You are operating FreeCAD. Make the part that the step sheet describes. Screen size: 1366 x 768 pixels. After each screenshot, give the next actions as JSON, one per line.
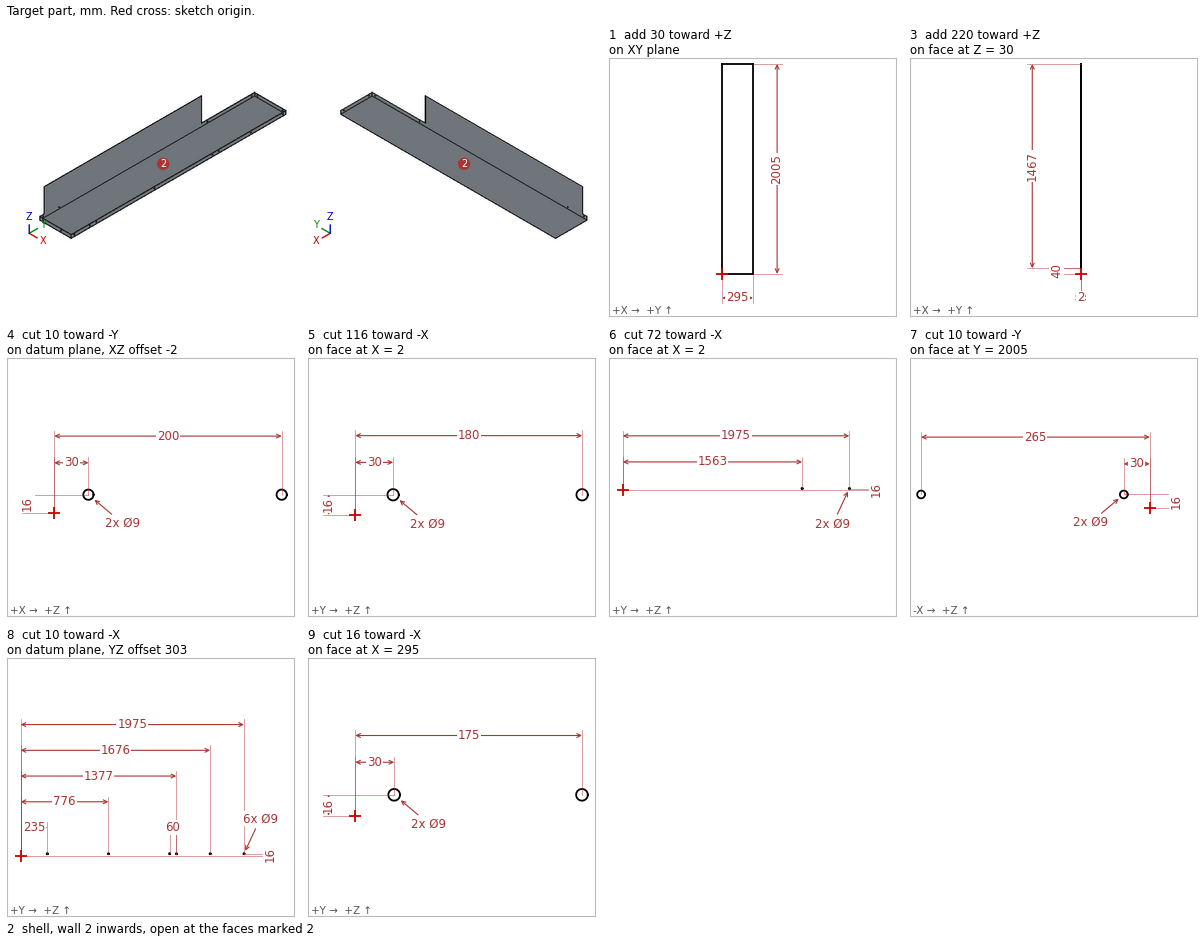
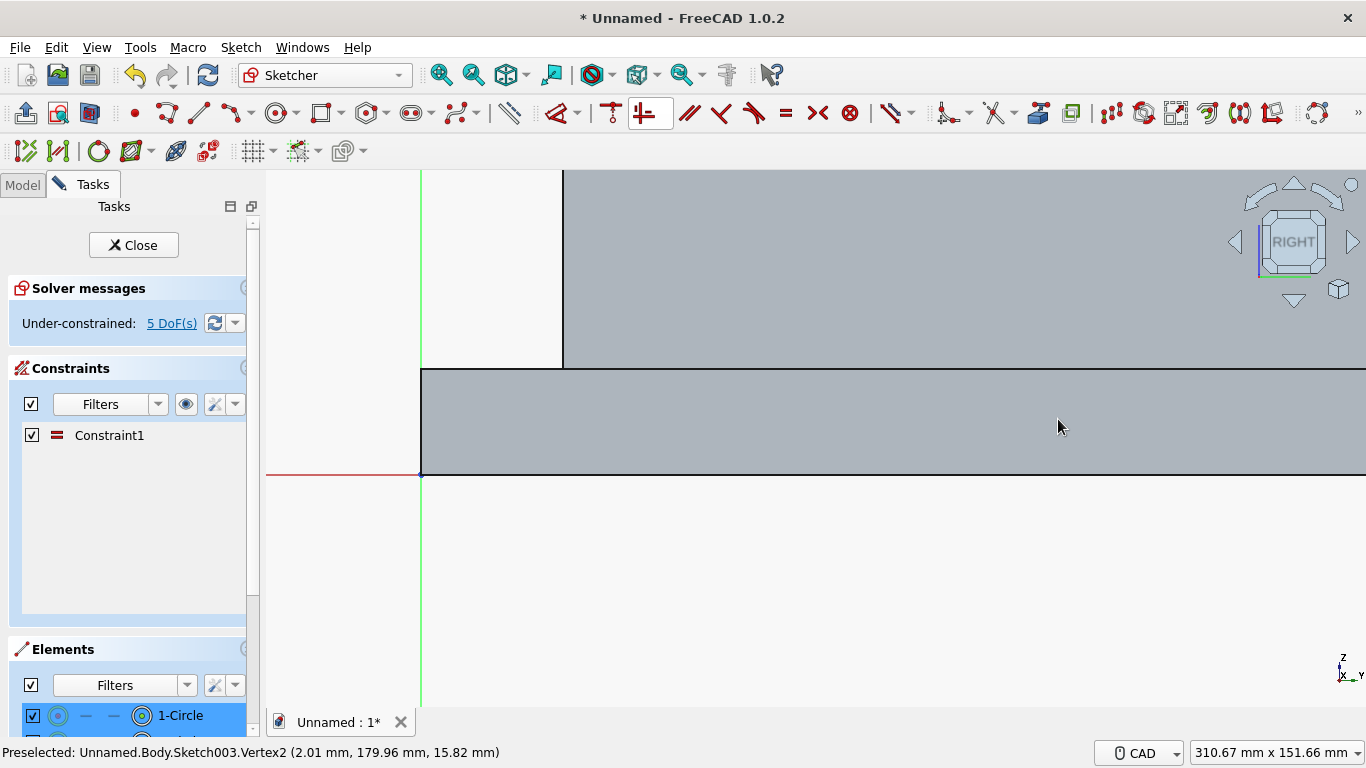
{"action": "key", "text": "h"}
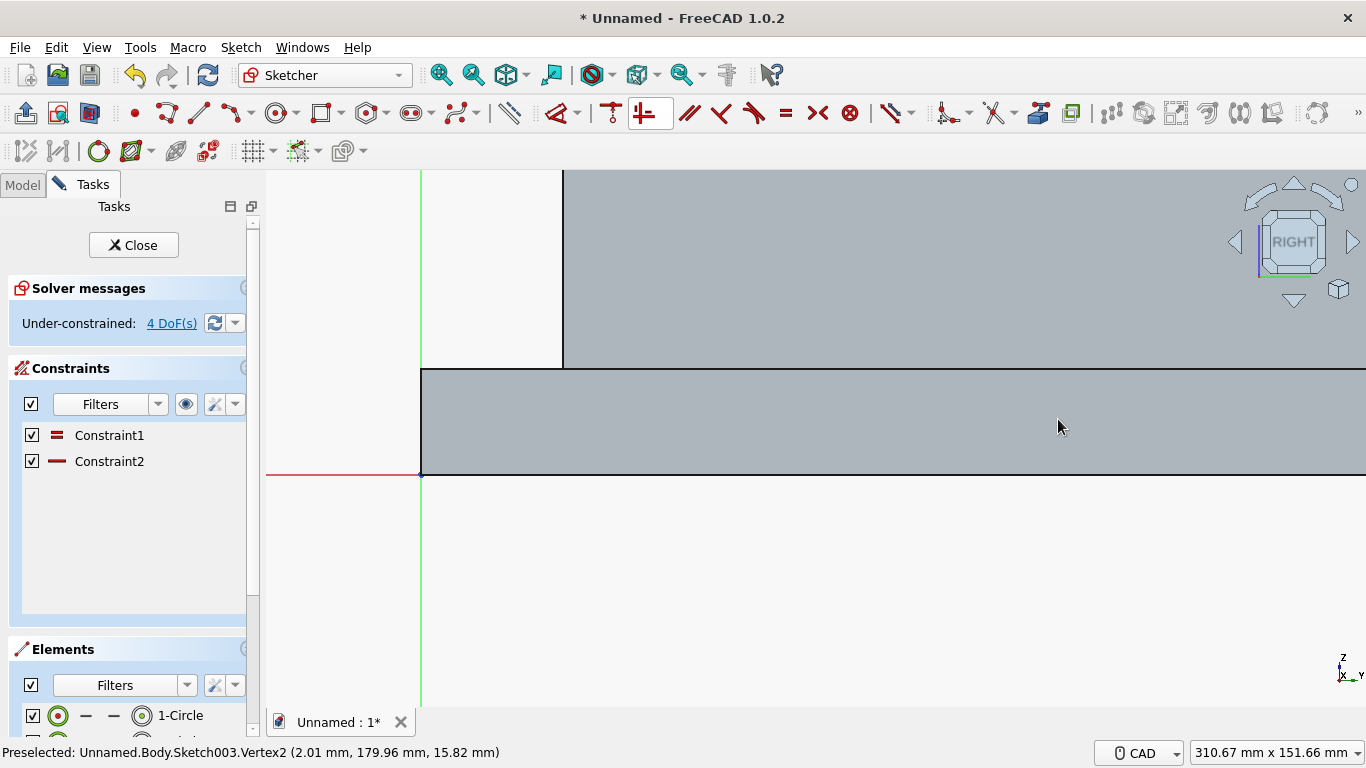
{"action": "left_click", "coordinate": [556, 114]}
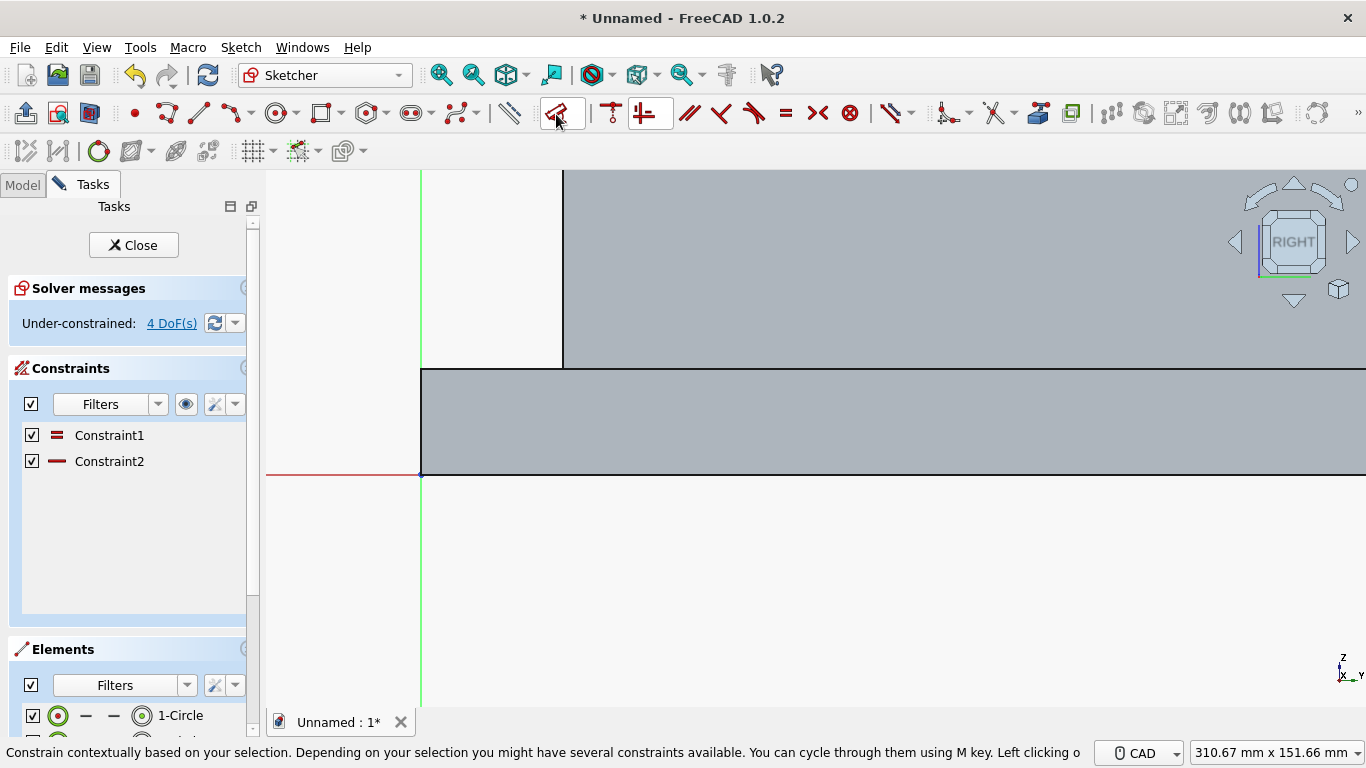
{"action": "scroll", "coordinate": [539, 407], "scroll_direction": "up", "scroll_amount": 2}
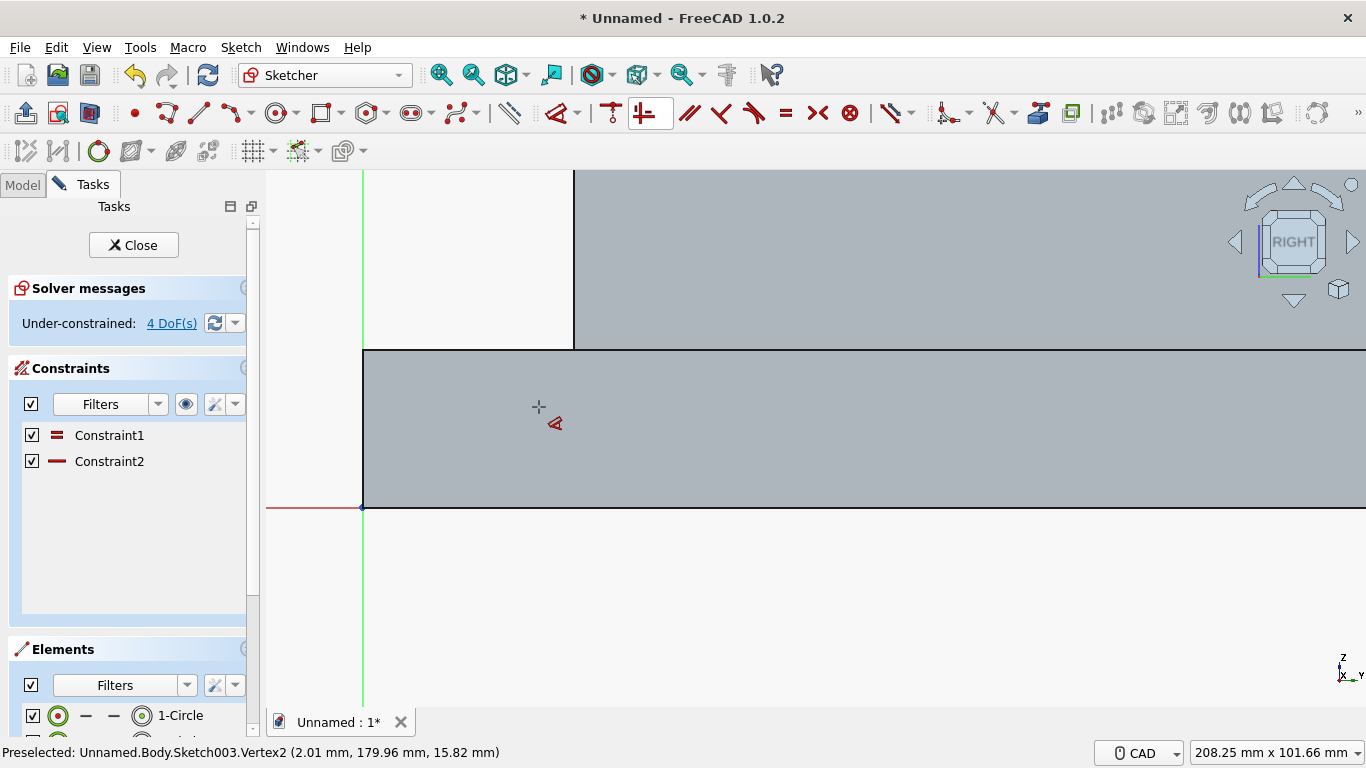
{"action": "left_click", "coordinate": [539, 407]}
{"action": "left_click", "coordinate": [562, 384]}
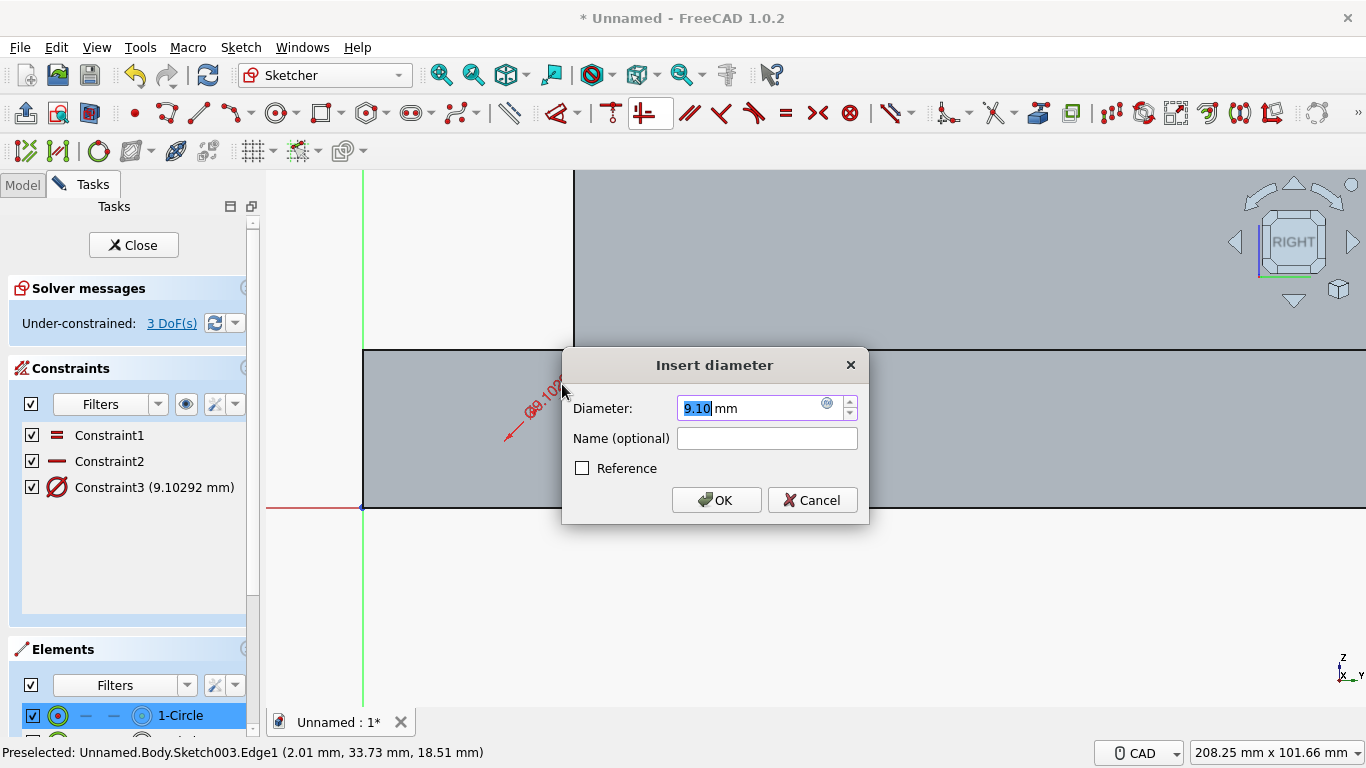
{"action": "type", "text": "9"}
{"action": "key", "text": "Return"}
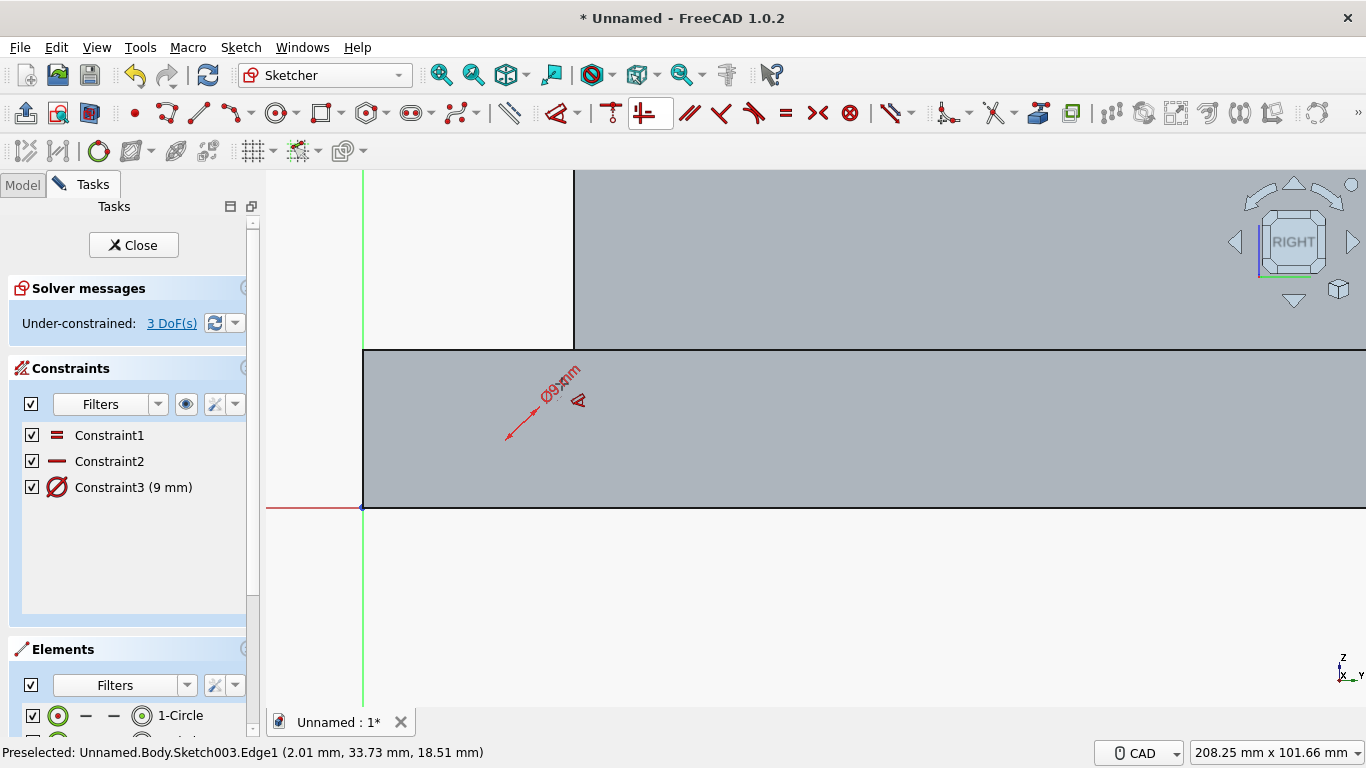
{"action": "left_click", "coordinate": [522, 424]}
{"action": "left_click", "coordinate": [442, 542]}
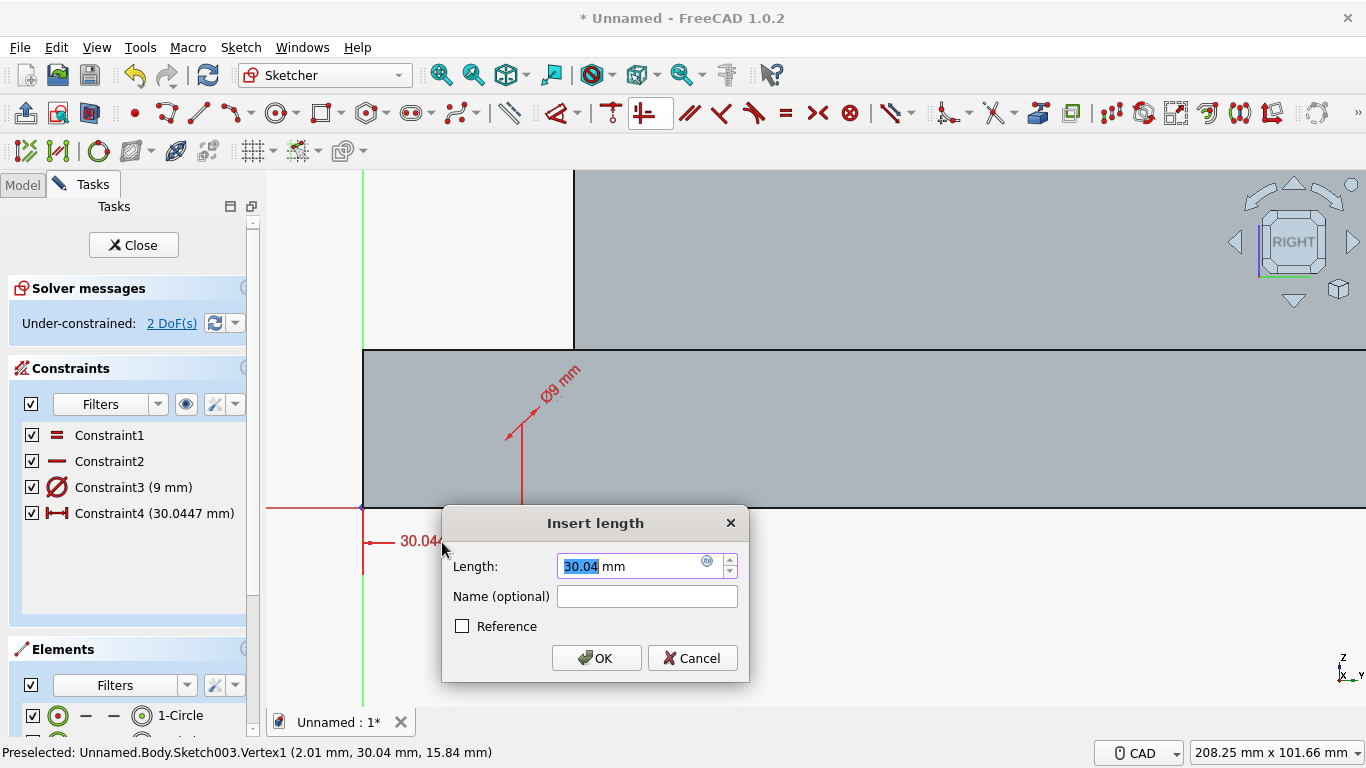
{"action": "type", "text": "30"}
{"action": "key", "text": "Return"}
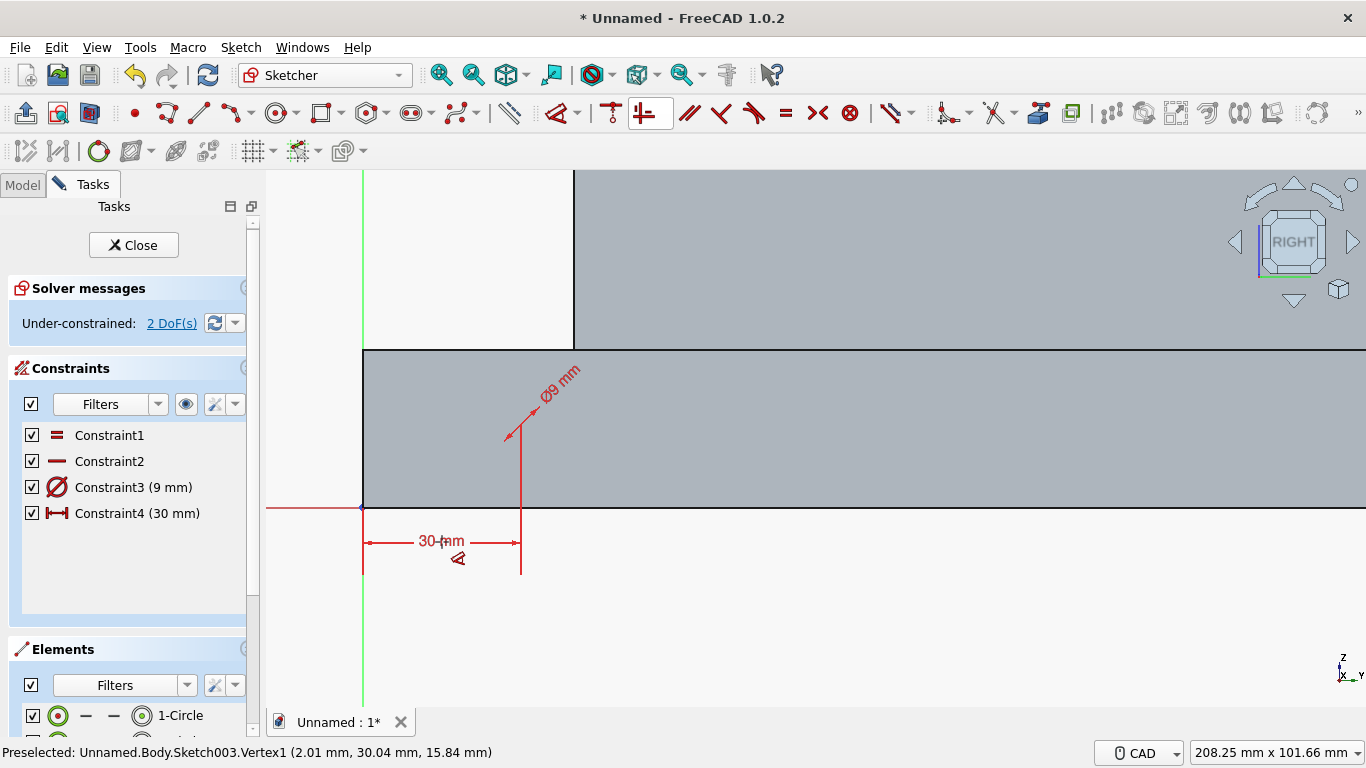
{"action": "left_click", "coordinate": [521, 424]}
{"action": "left_click", "coordinate": [329, 466]}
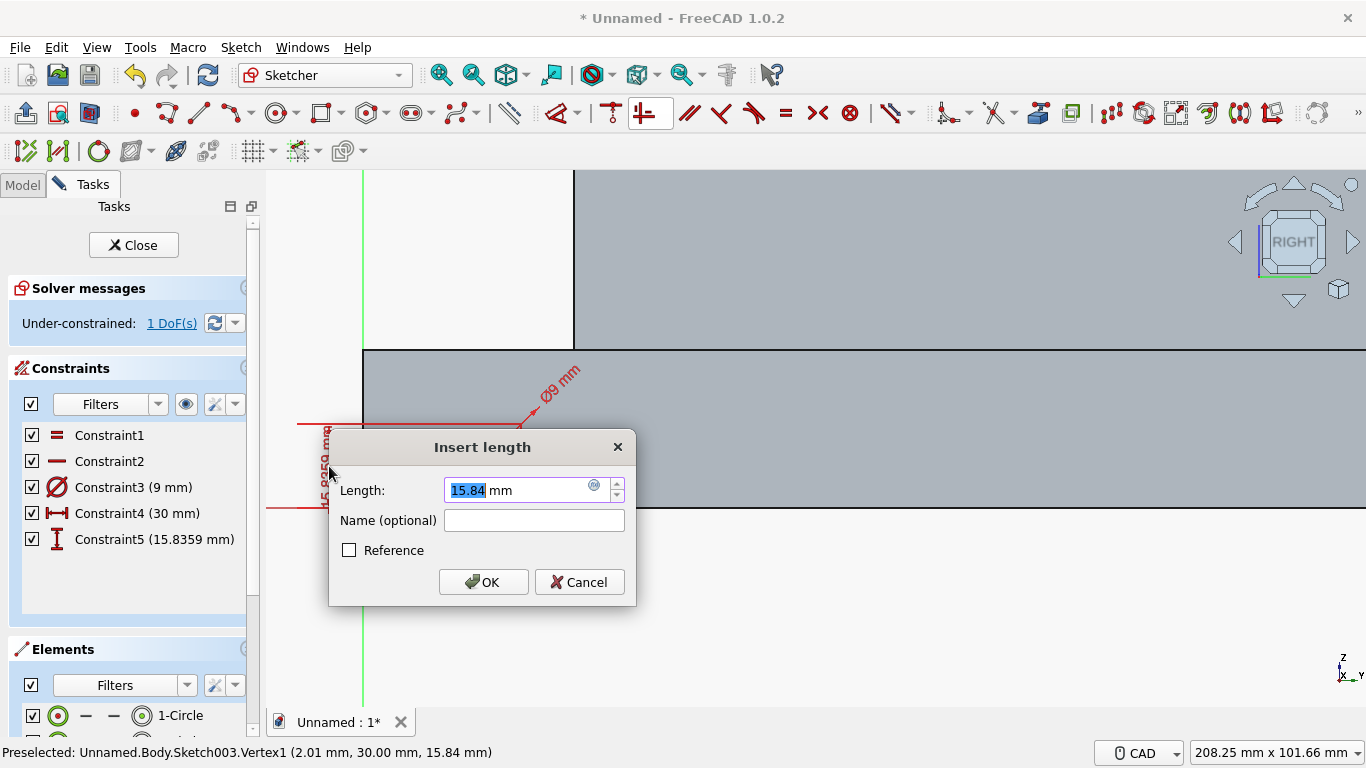
{"action": "type", "text": "16"}
{"action": "key", "text": "Return"}